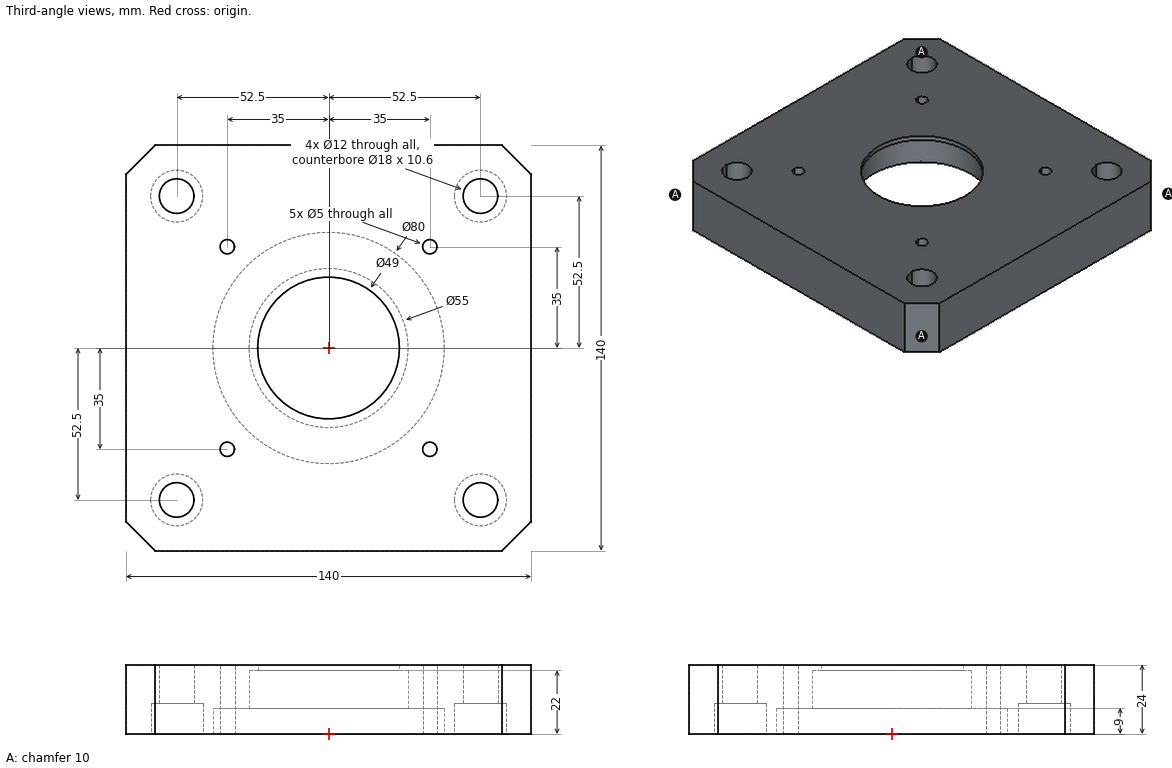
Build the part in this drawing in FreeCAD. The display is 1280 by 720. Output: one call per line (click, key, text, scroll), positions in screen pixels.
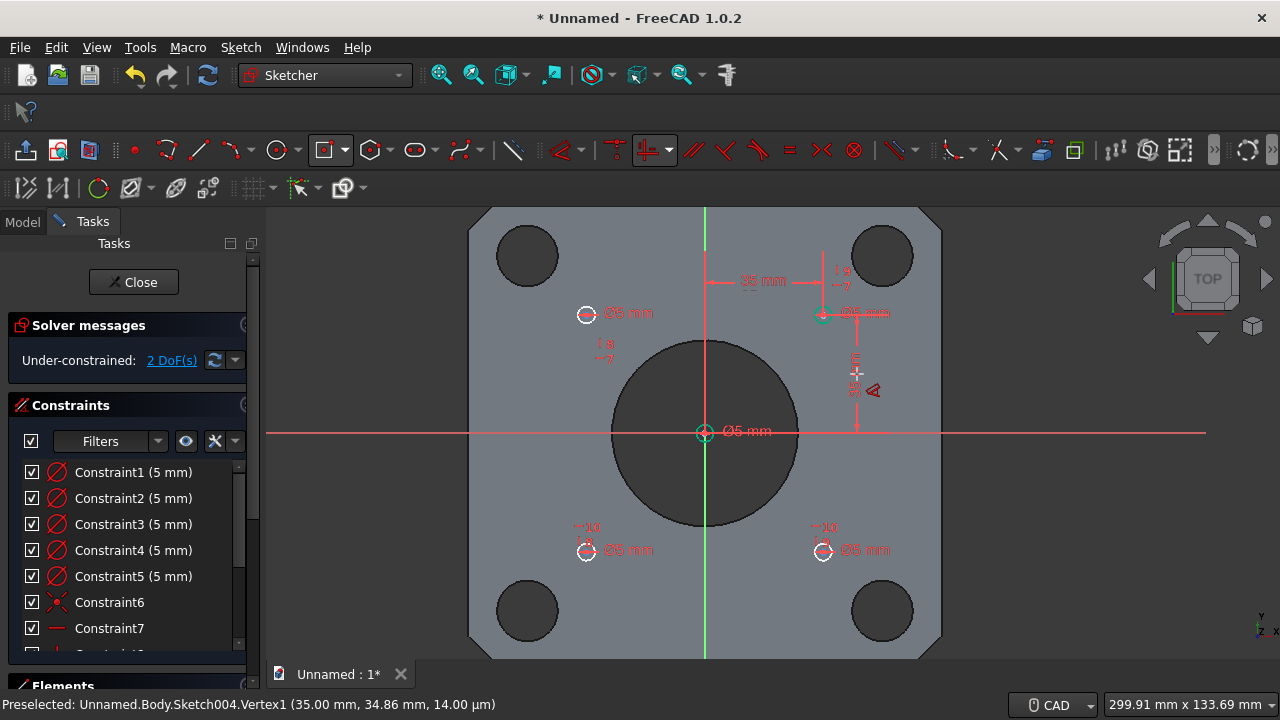
click(586, 315)
click(646, 281)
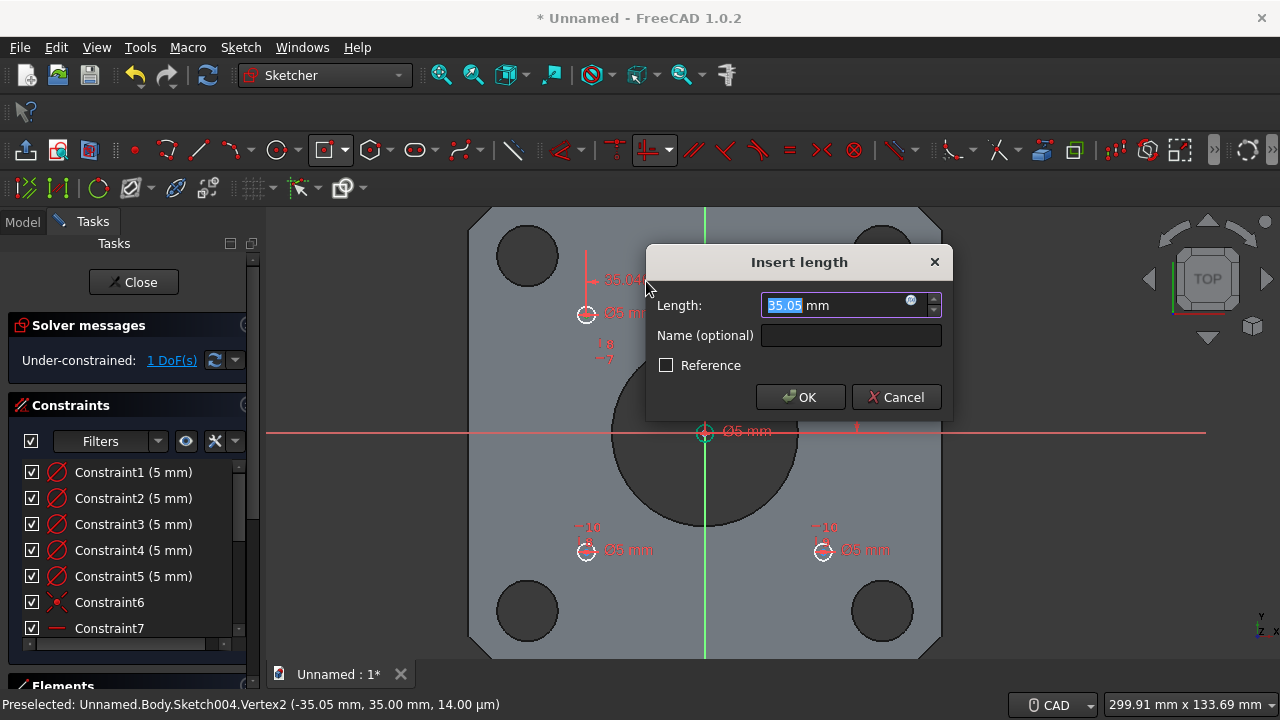
text(35)
key(Return)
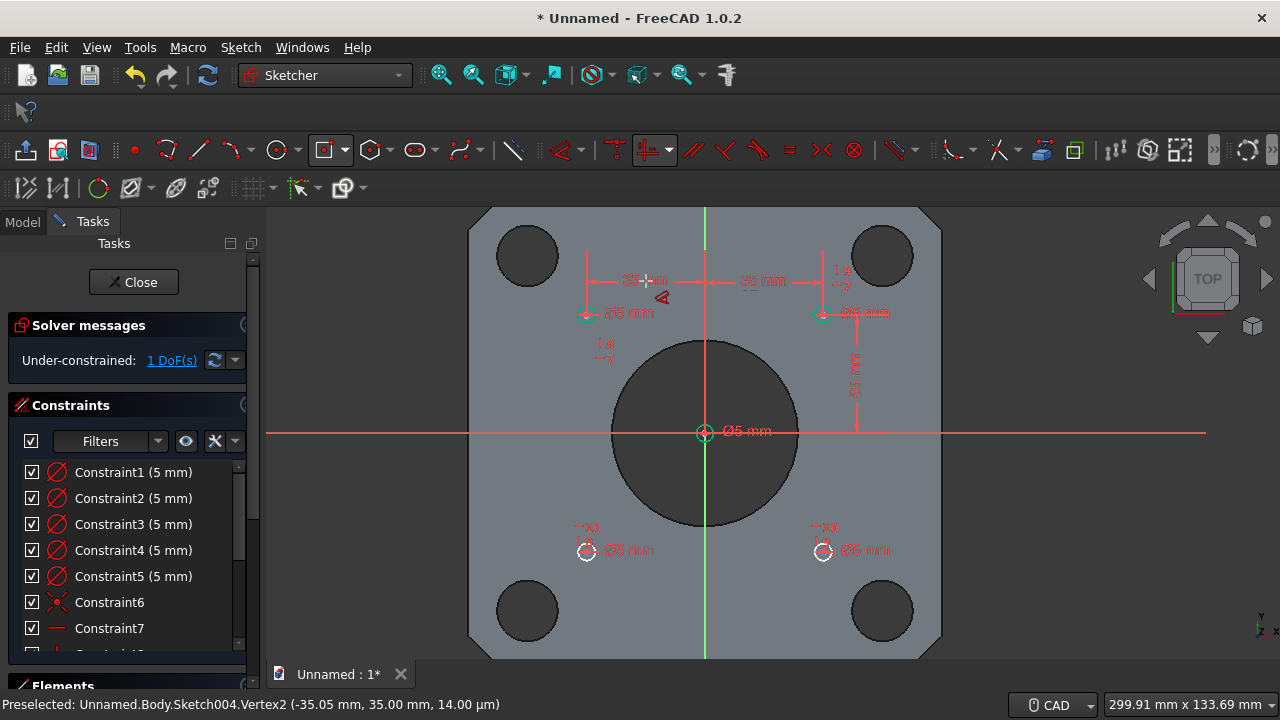
click(587, 552)
click(553, 493)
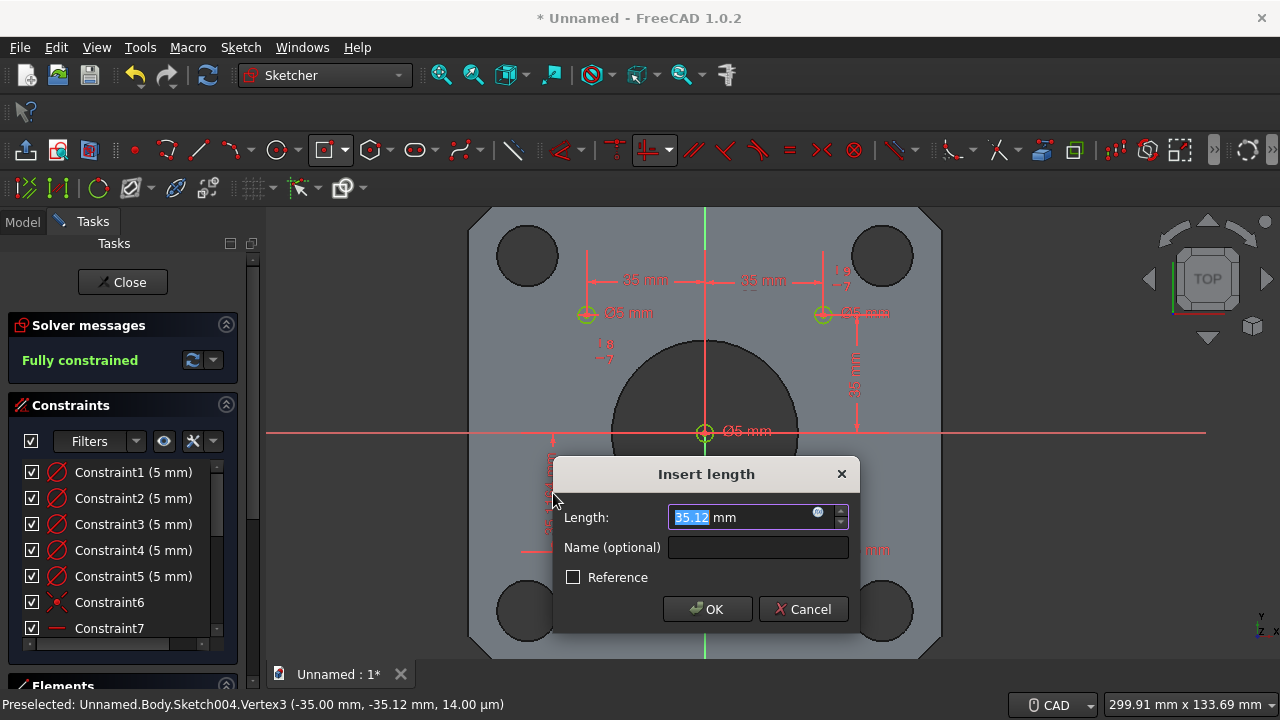
text(35)
key(Return)
key(Escape)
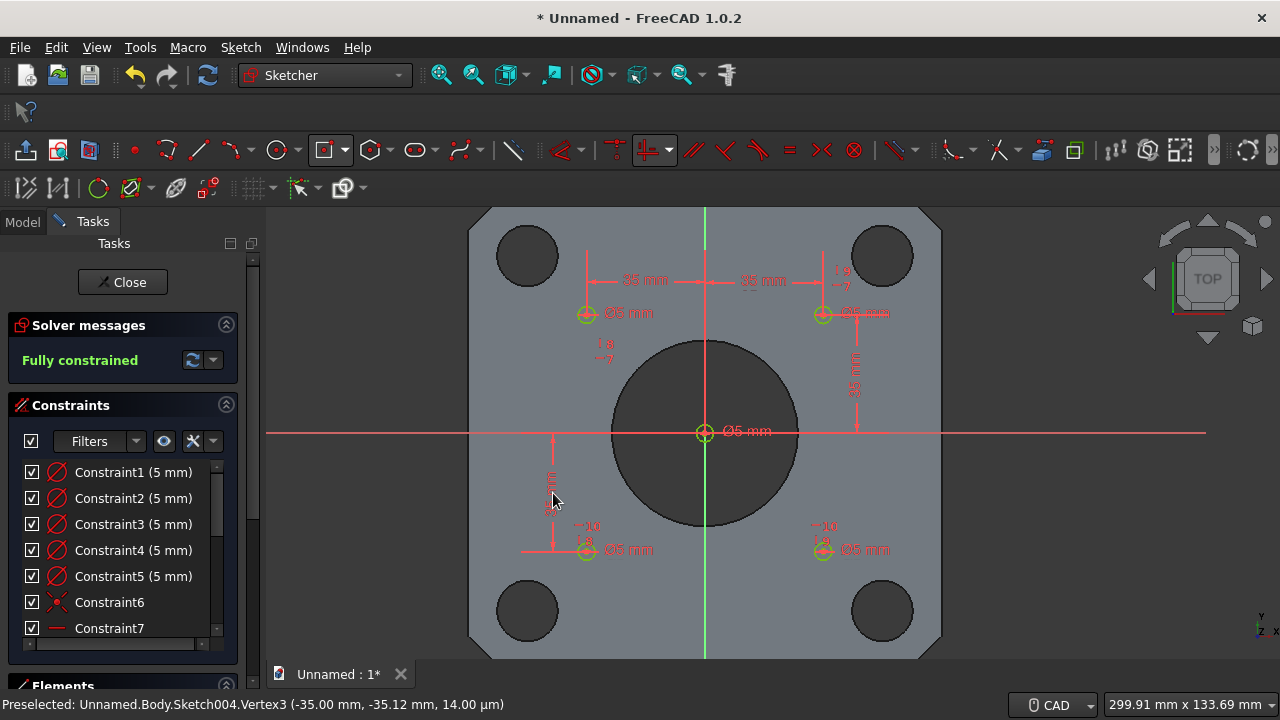
click(123, 282)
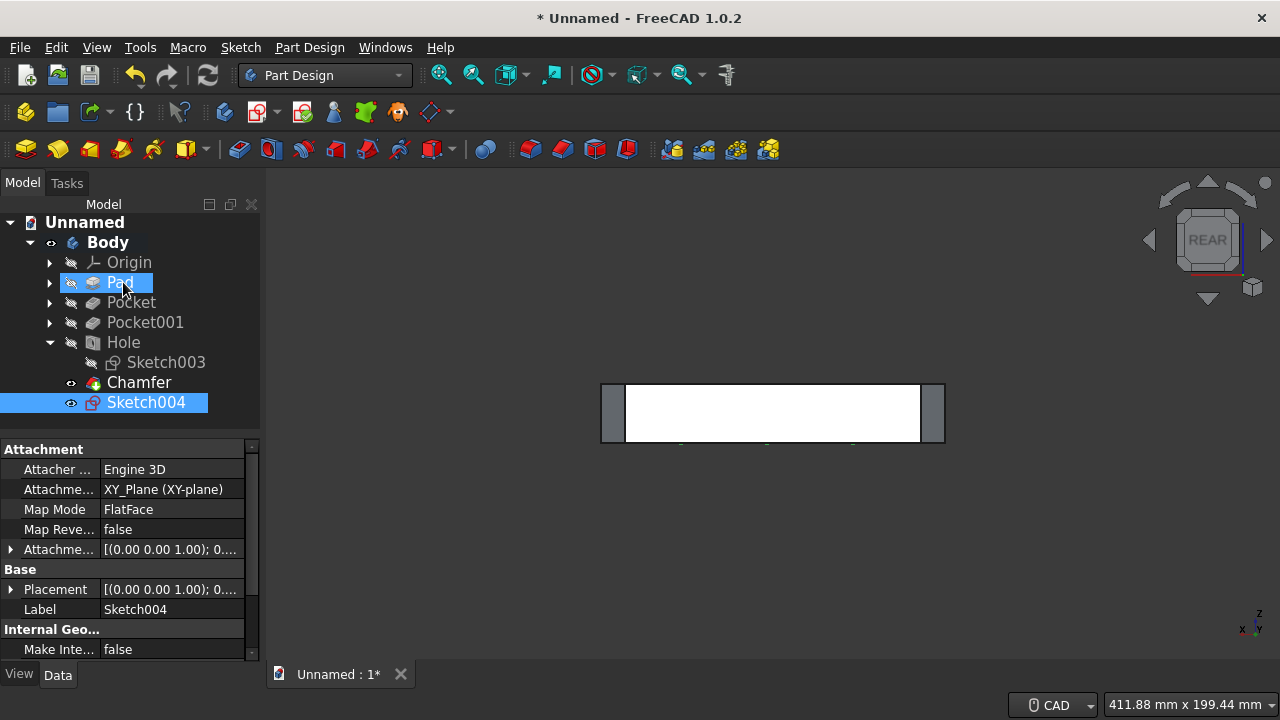
click(272, 150)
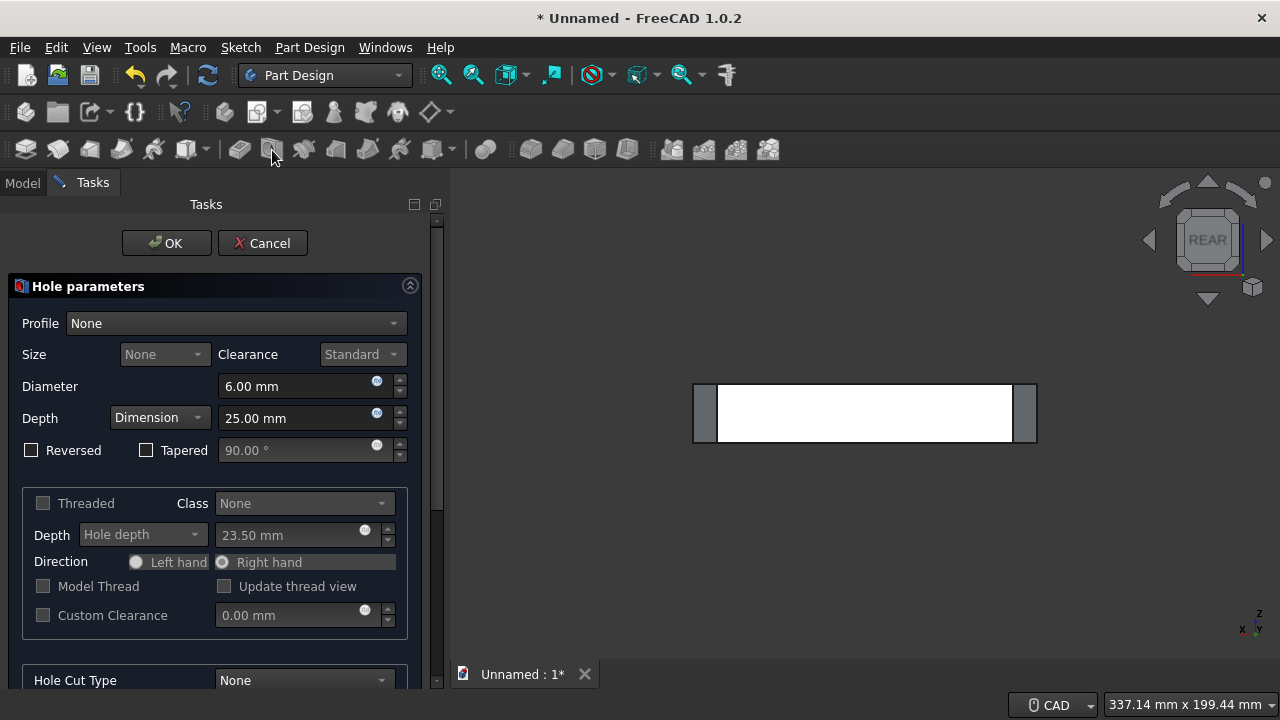
triple_click(305, 386)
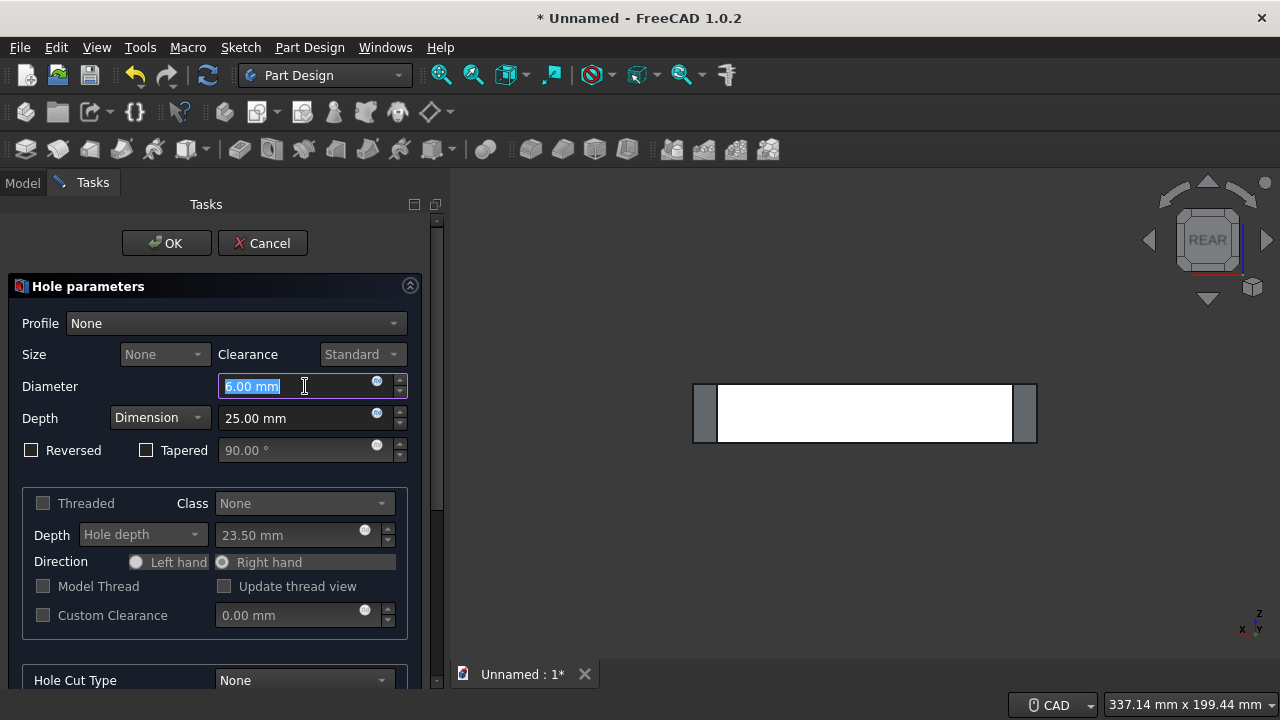
text(5)
key(Tab)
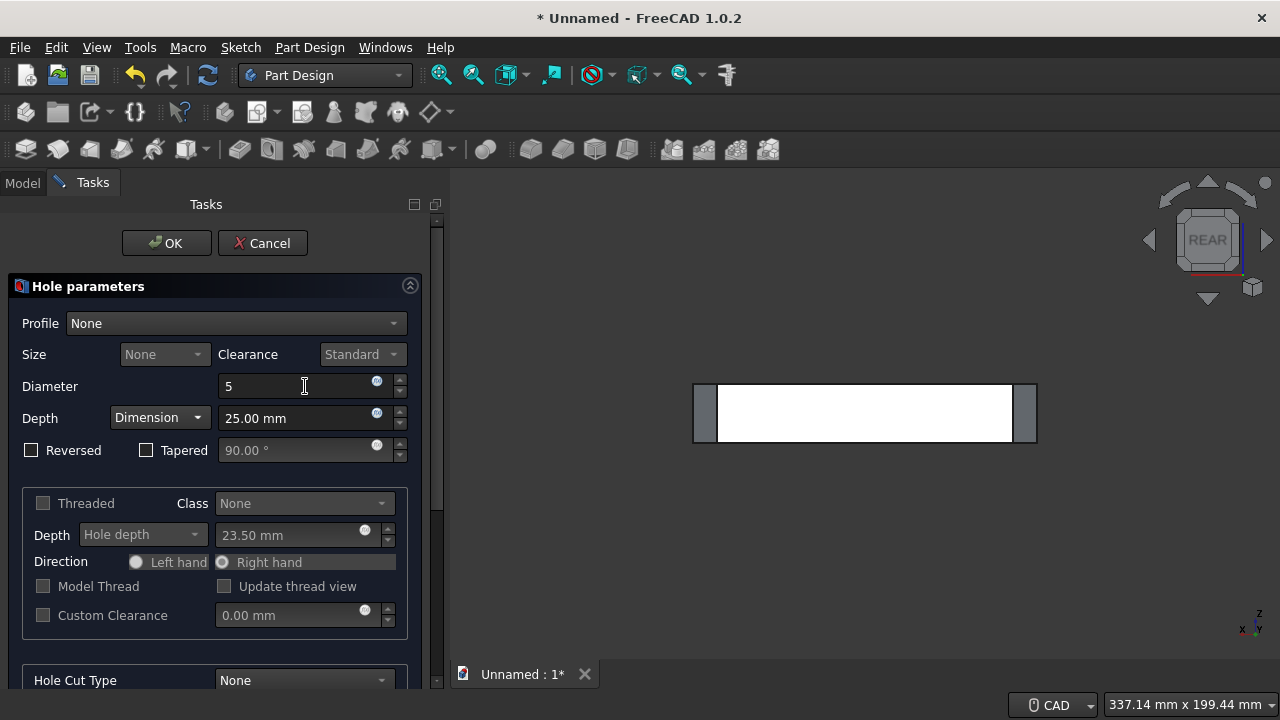
click(161, 418)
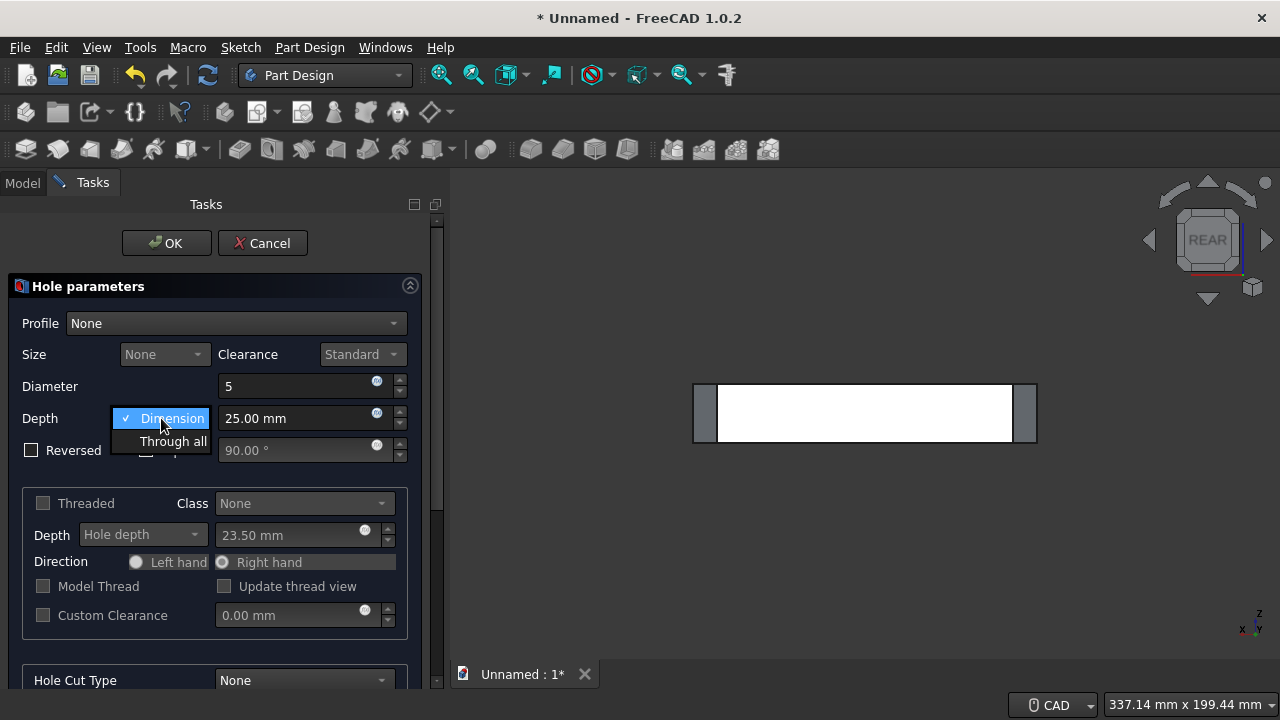
click(160, 442)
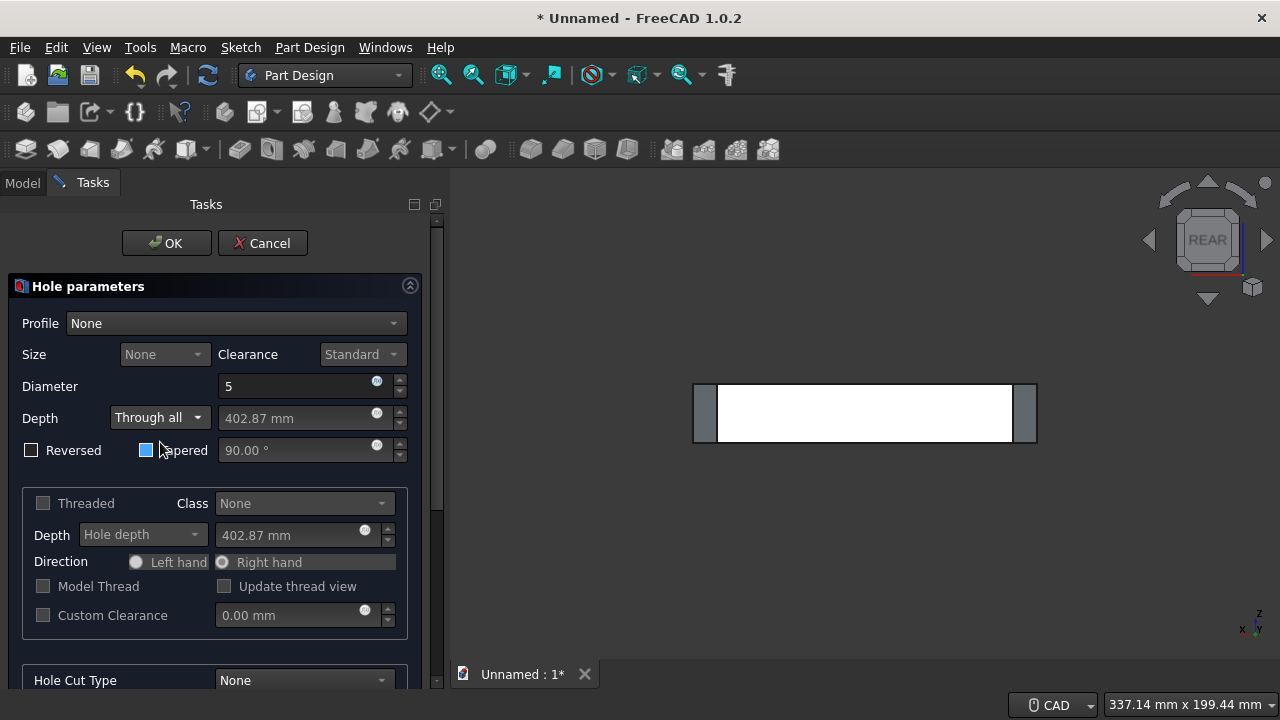
click(30, 450)